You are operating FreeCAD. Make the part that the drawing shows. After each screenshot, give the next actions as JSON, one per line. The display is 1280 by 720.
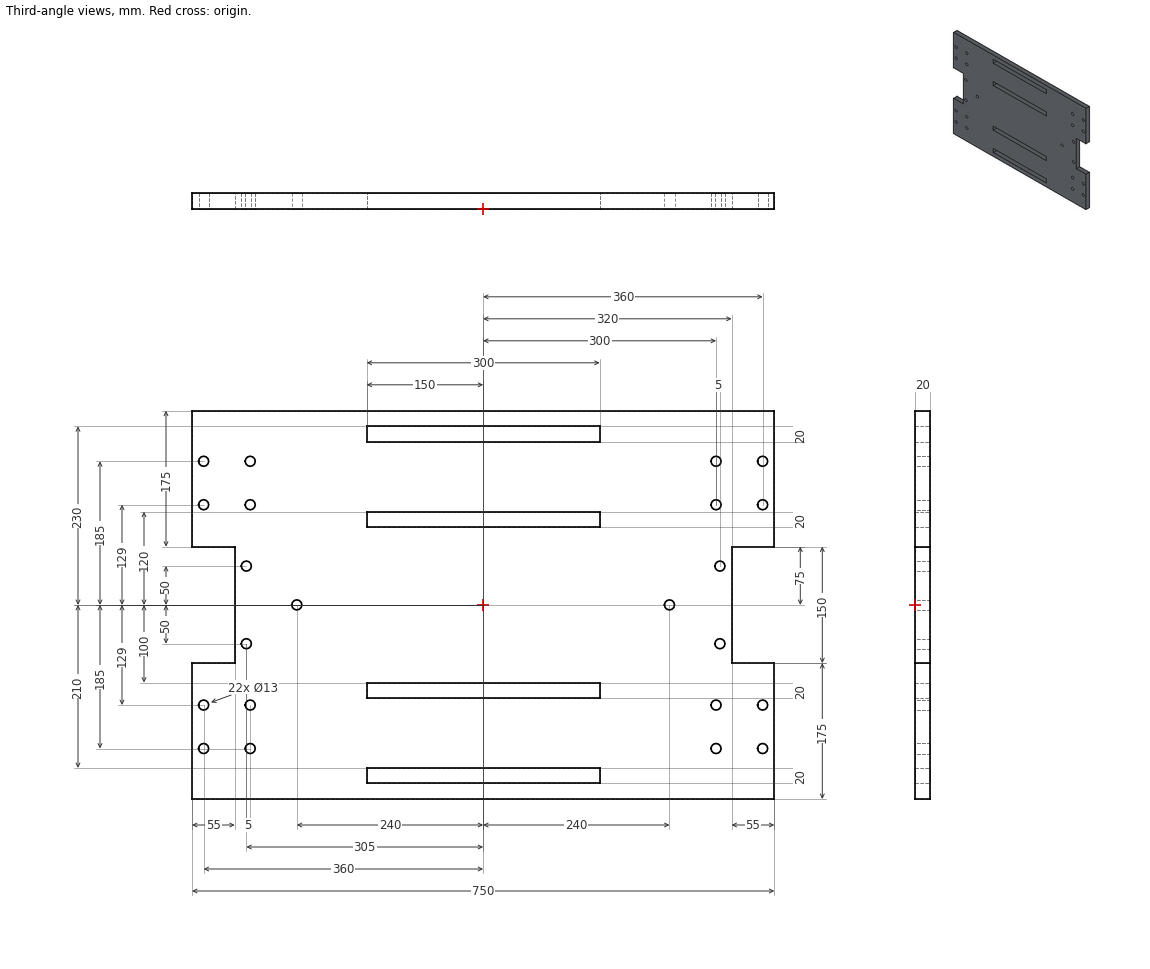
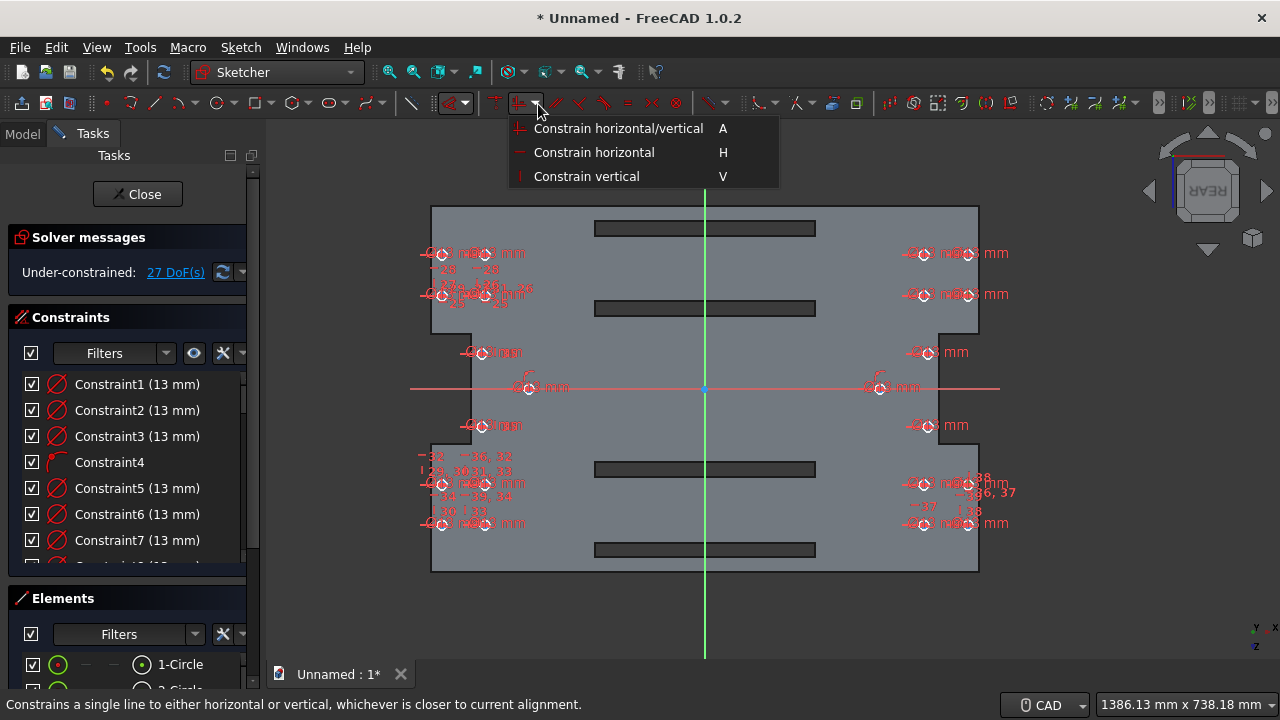
{"action": "left_click", "coordinate": [644, 176]}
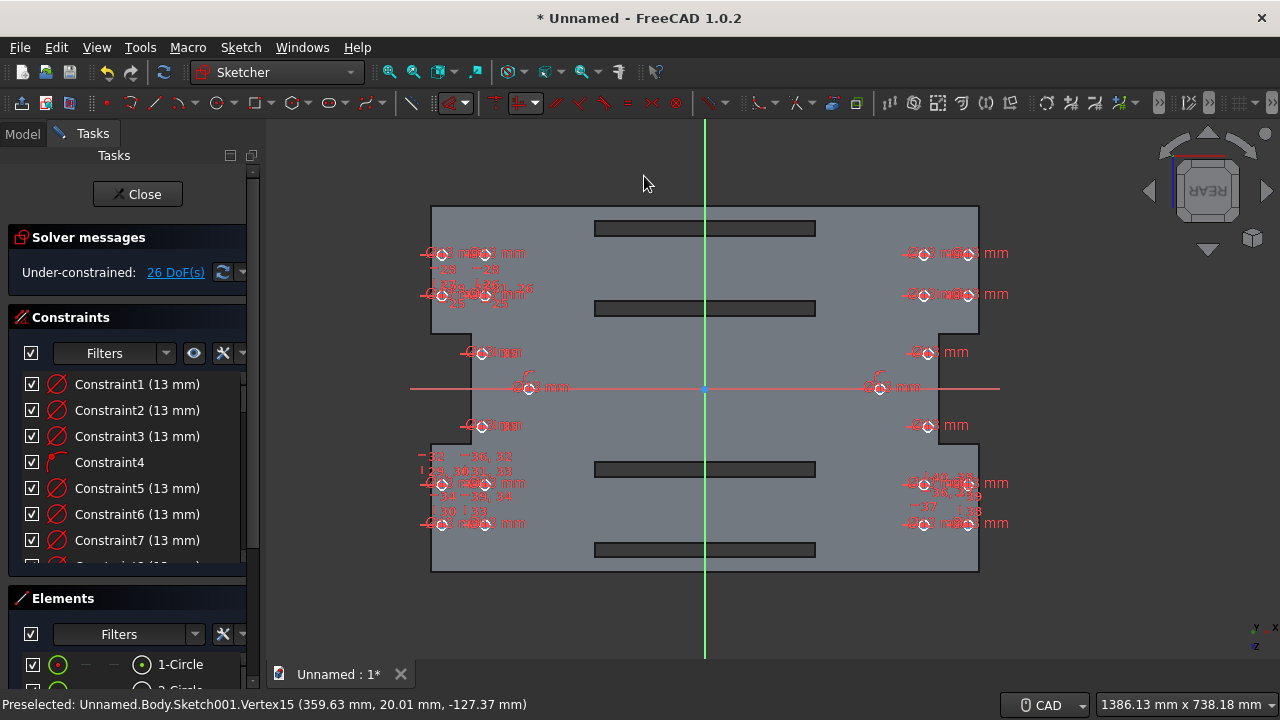
{"action": "left_click", "coordinate": [485, 296]}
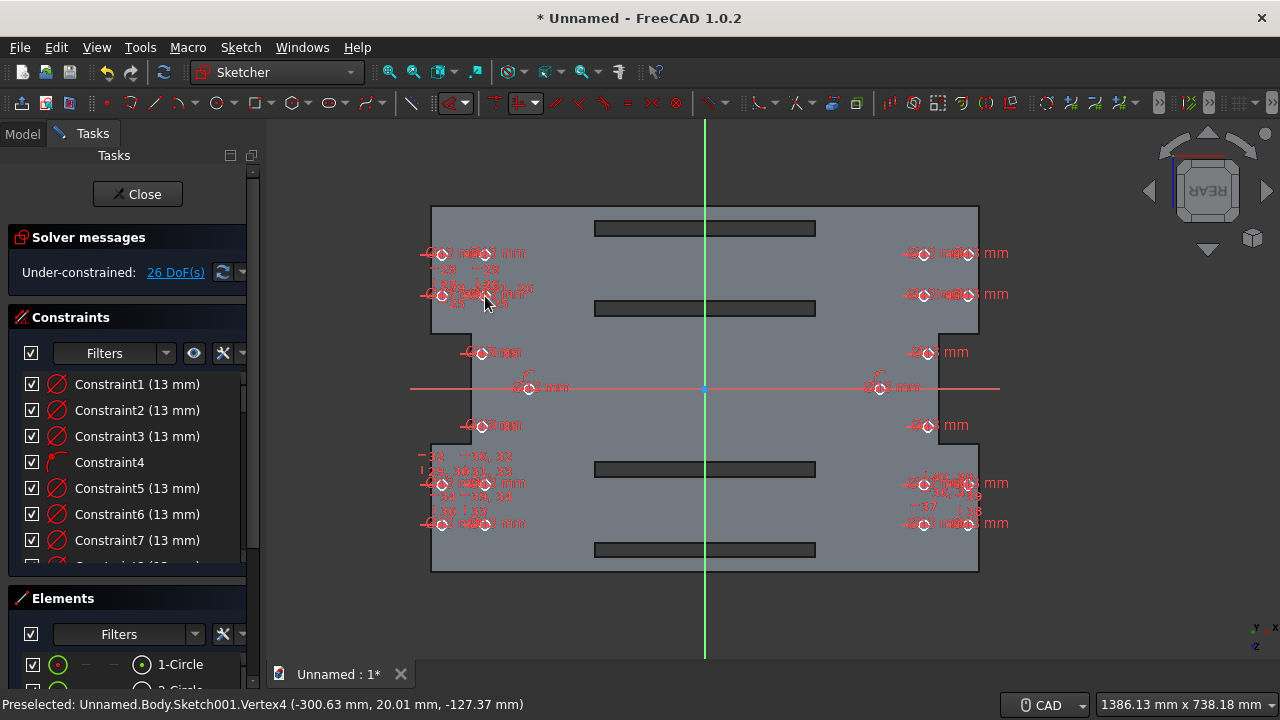
{"action": "left_click", "coordinate": [968, 296]}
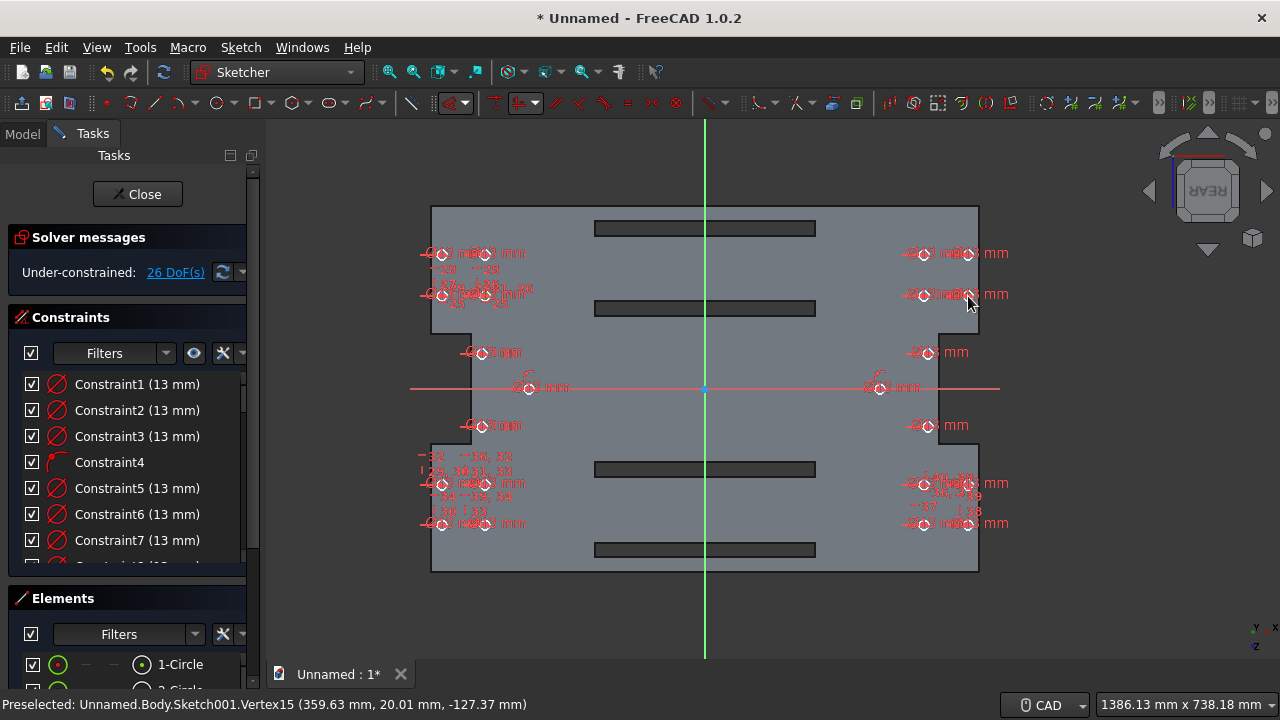
{"action": "left_click", "coordinate": [538, 104]}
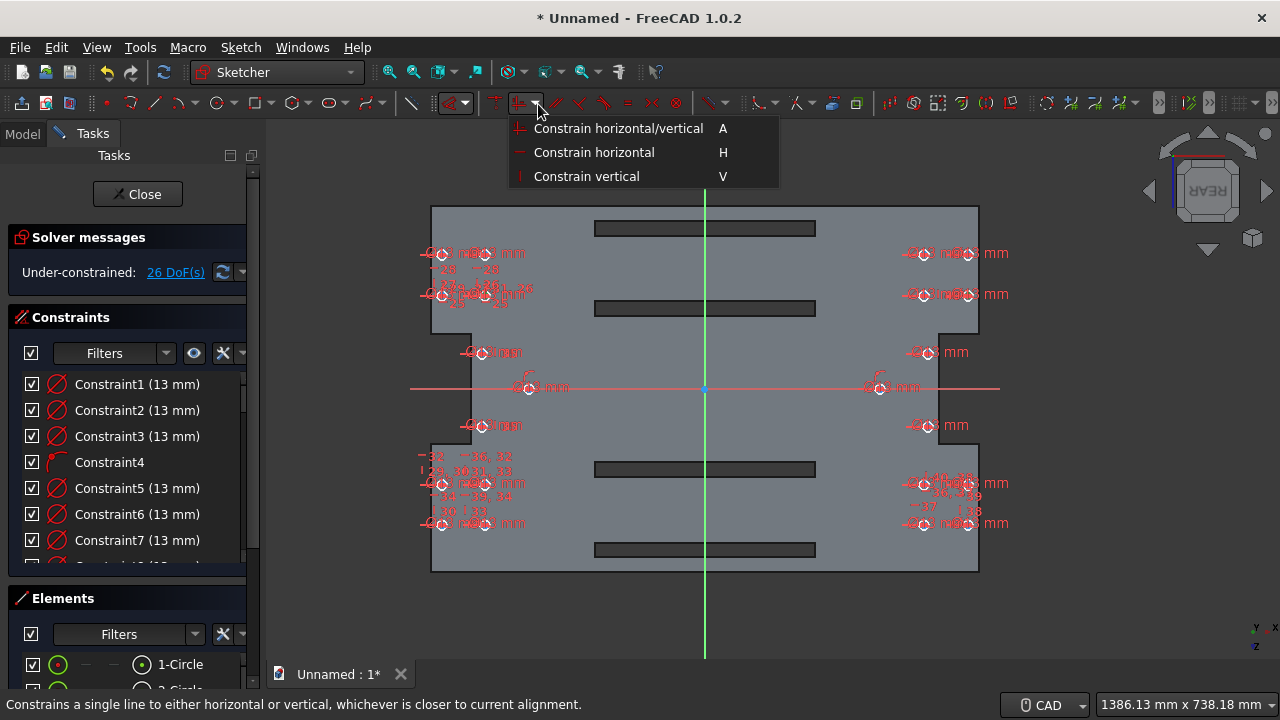
{"action": "left_click", "coordinate": [644, 152]}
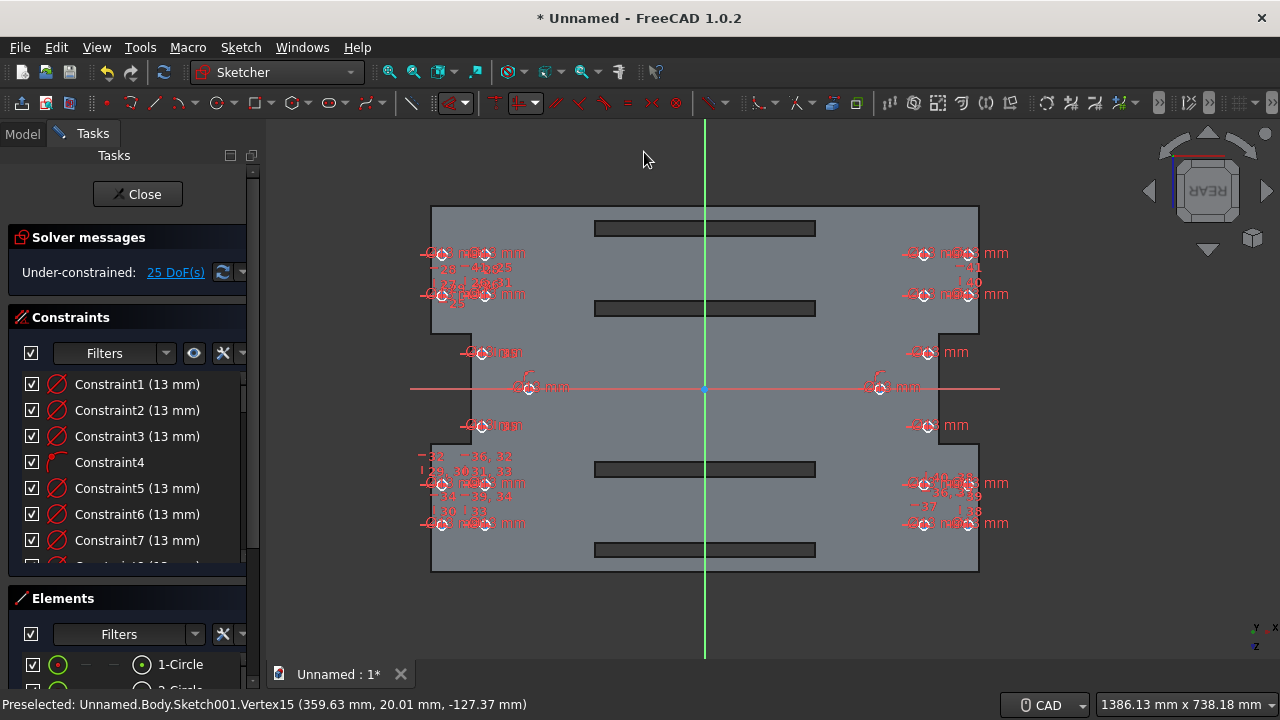
{"action": "left_click", "coordinate": [968, 296]}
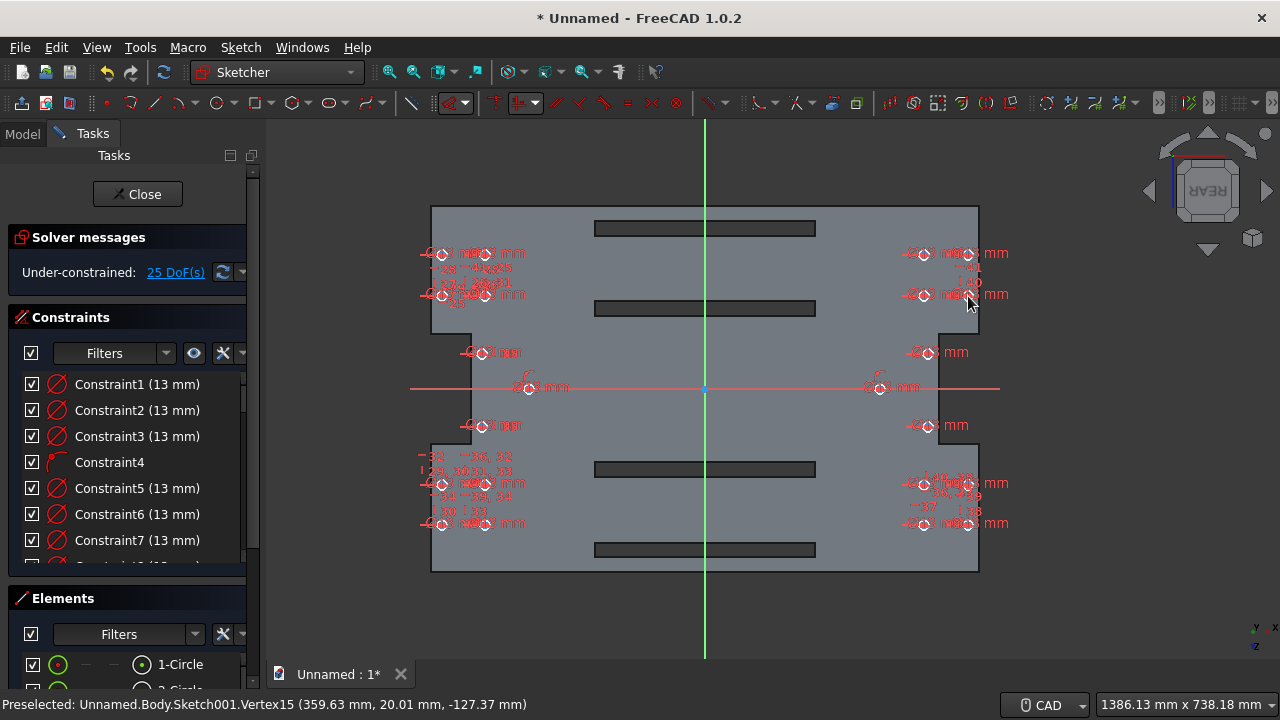
{"action": "left_click", "coordinate": [968, 255]}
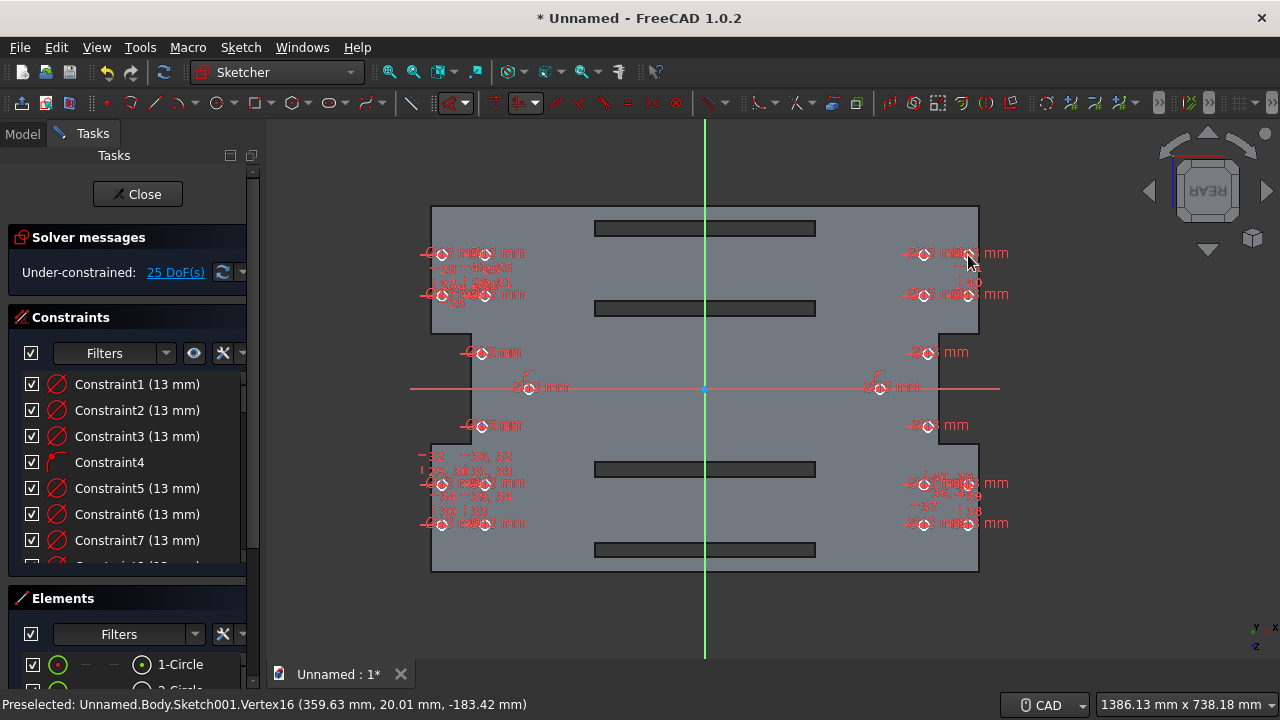
{"action": "left_click", "coordinate": [538, 104]}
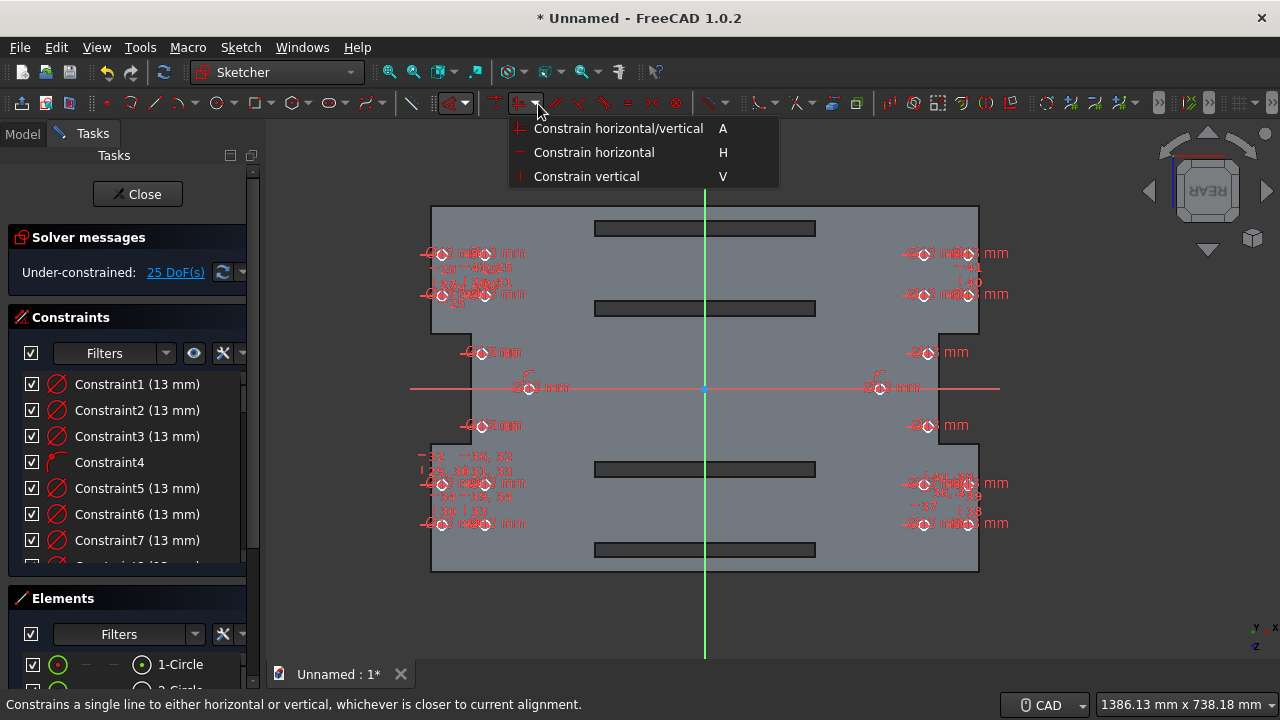
{"action": "left_click", "coordinate": [644, 176]}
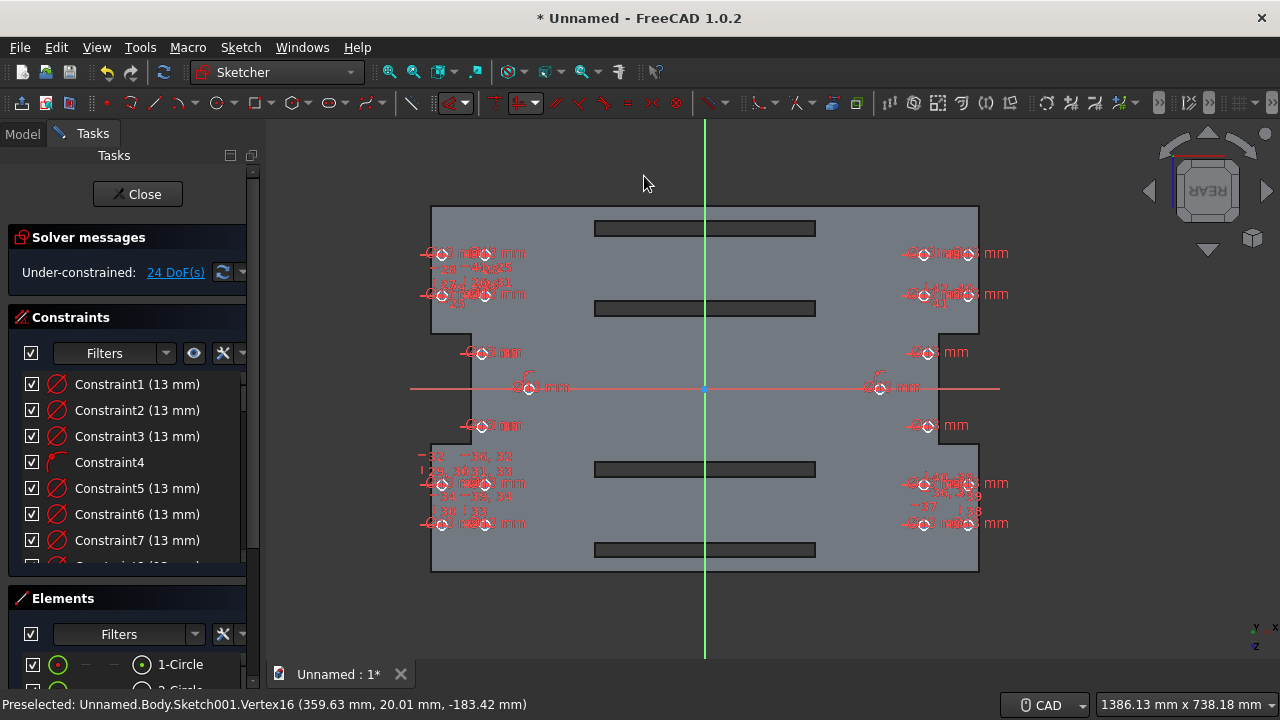
{"action": "left_click", "coordinate": [485, 255]}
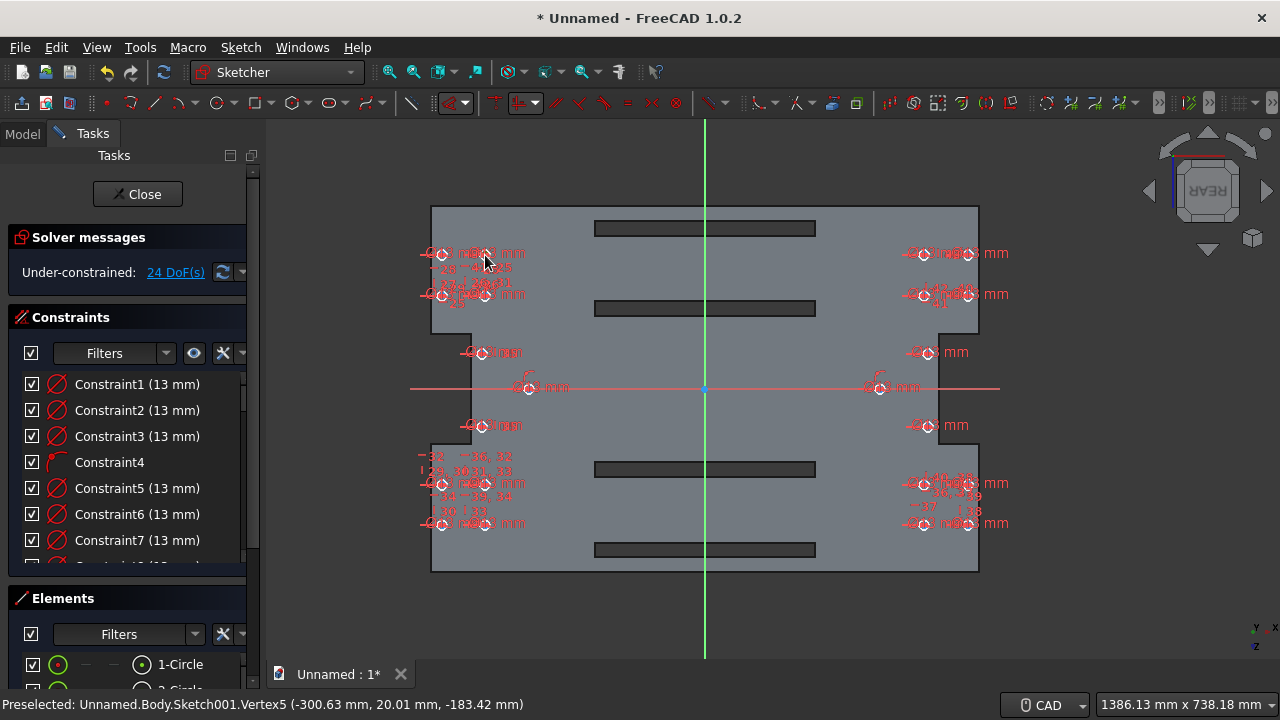
{"action": "left_click", "coordinate": [968, 255]}